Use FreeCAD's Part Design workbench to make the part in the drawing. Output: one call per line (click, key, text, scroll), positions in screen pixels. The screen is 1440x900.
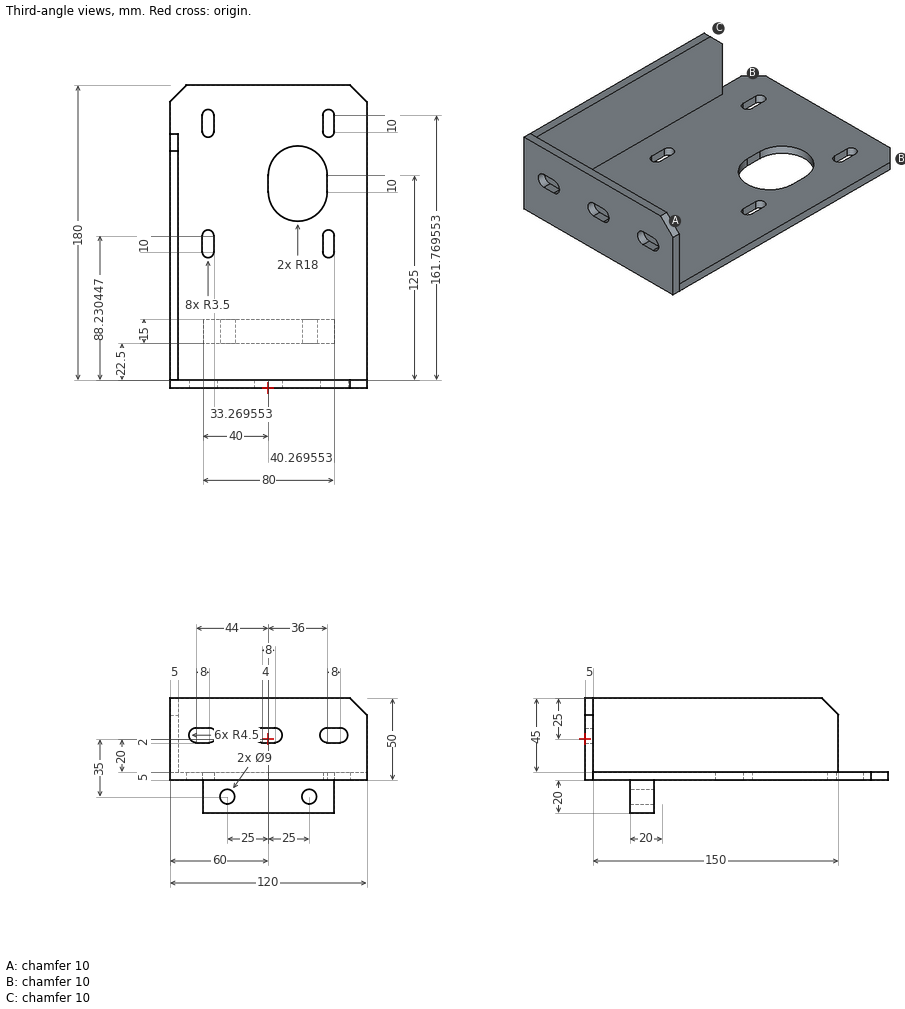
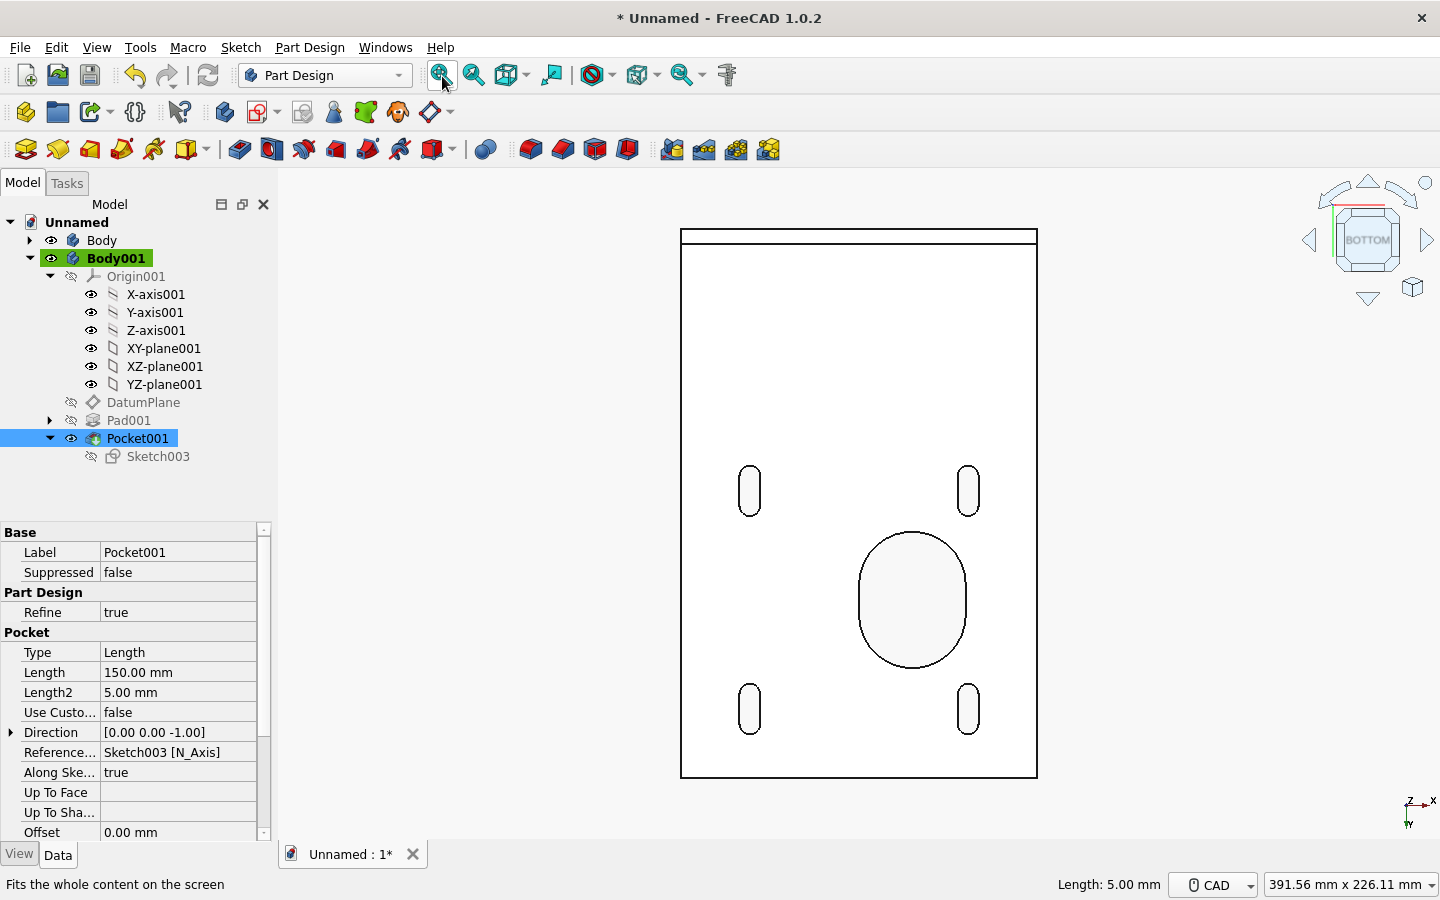
scroll(681, 777, up, 5)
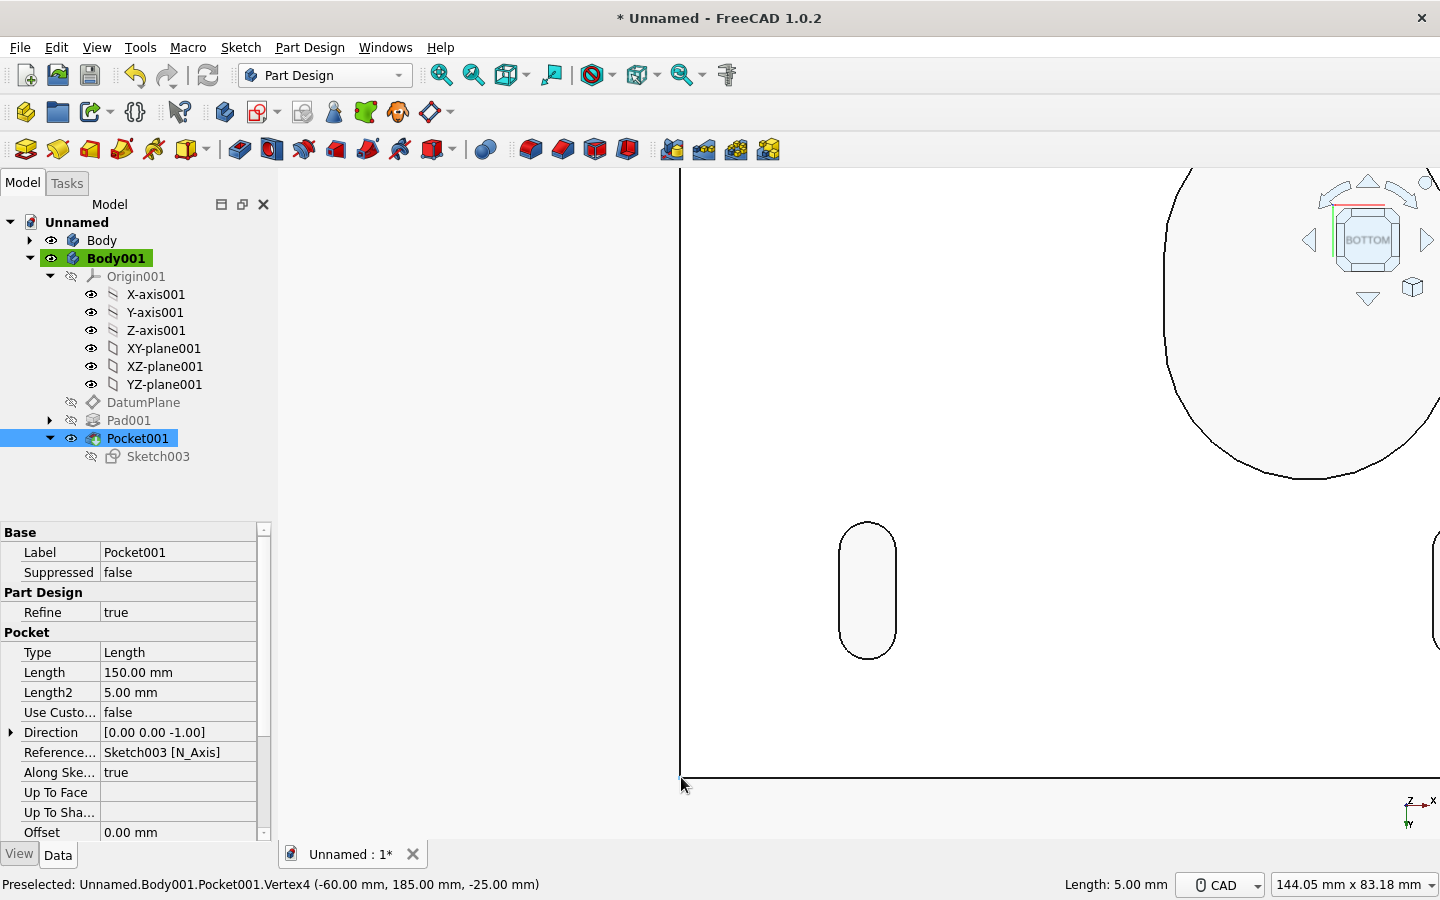
key(v)
key(f)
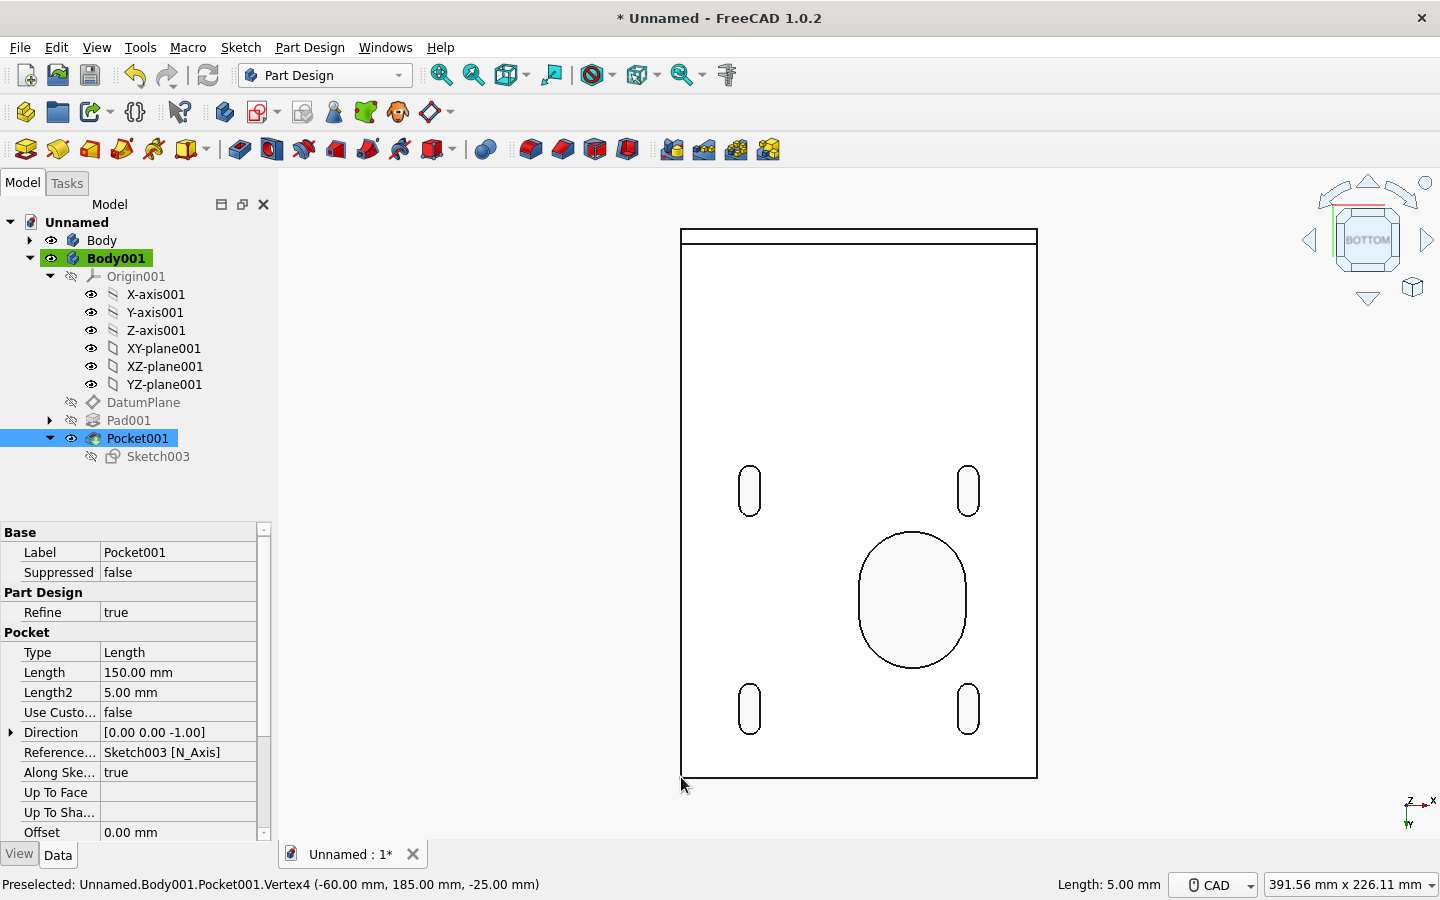
key(4)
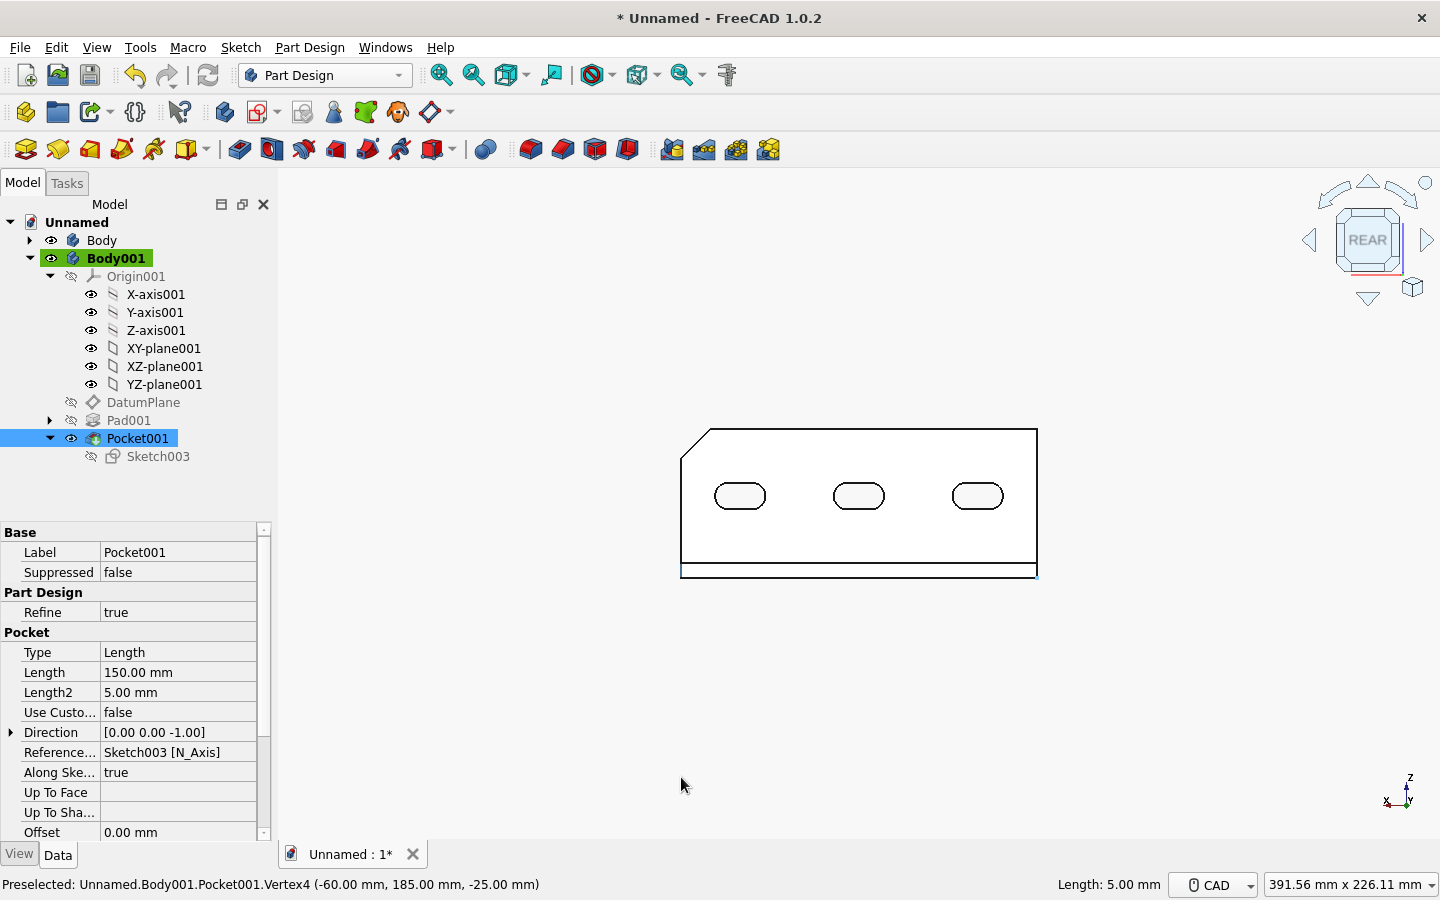
click(442, 76)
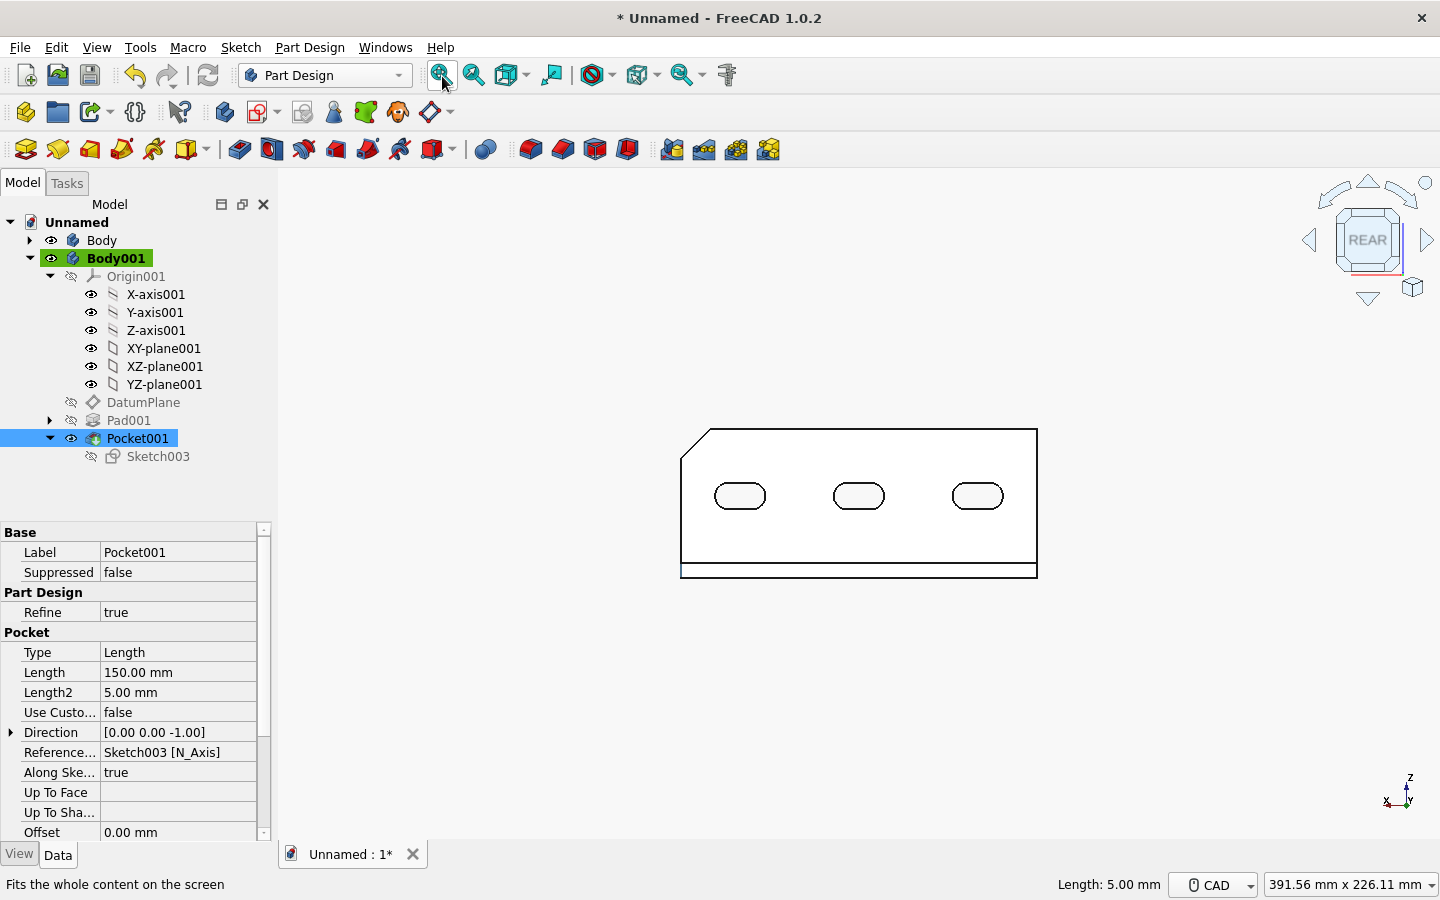
click(1037, 569, ctrl)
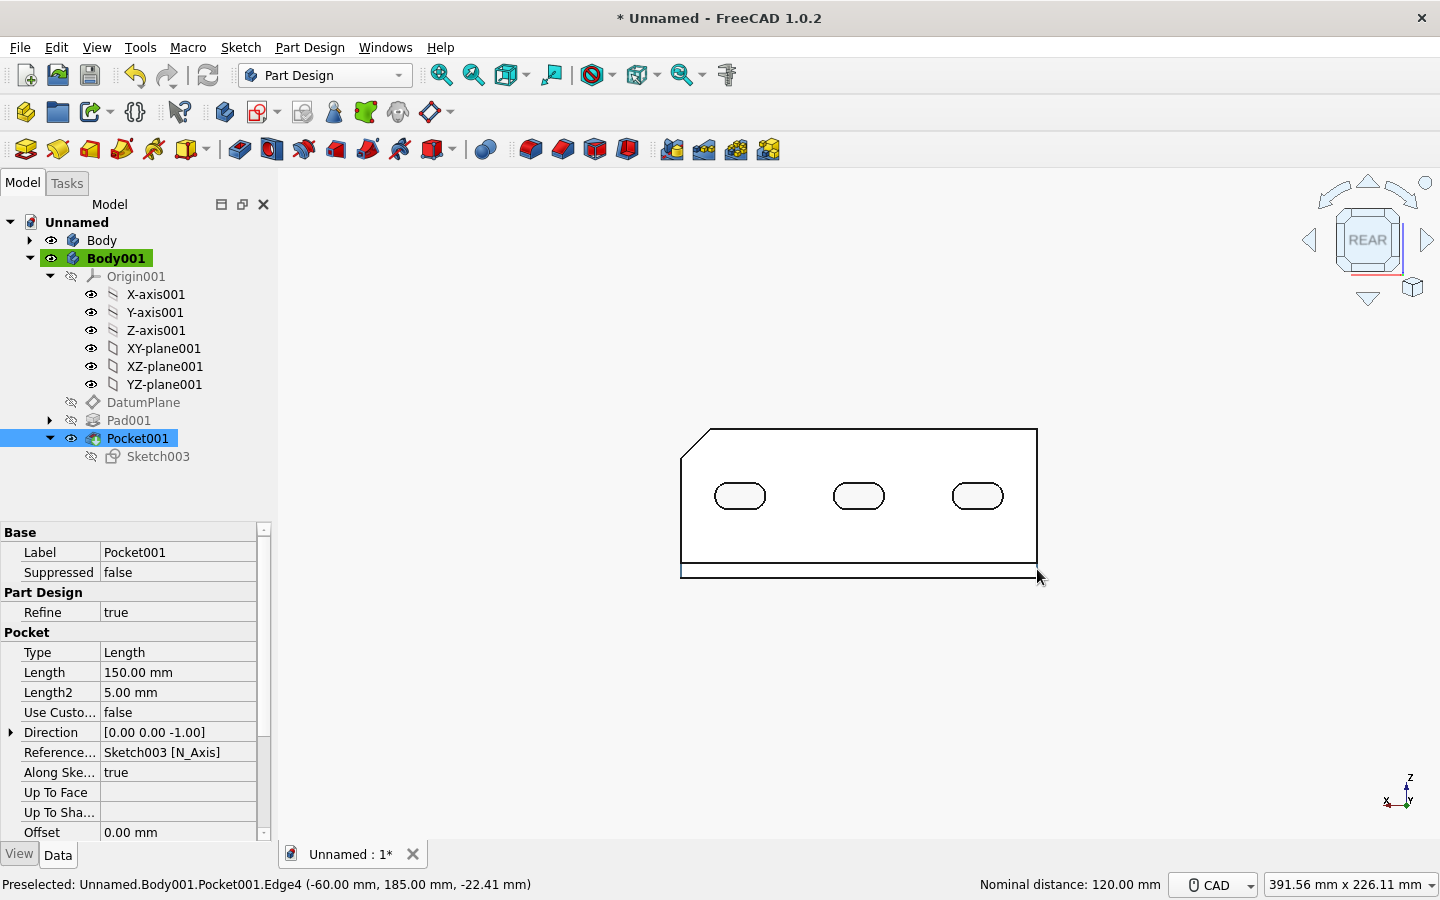
click(564, 150)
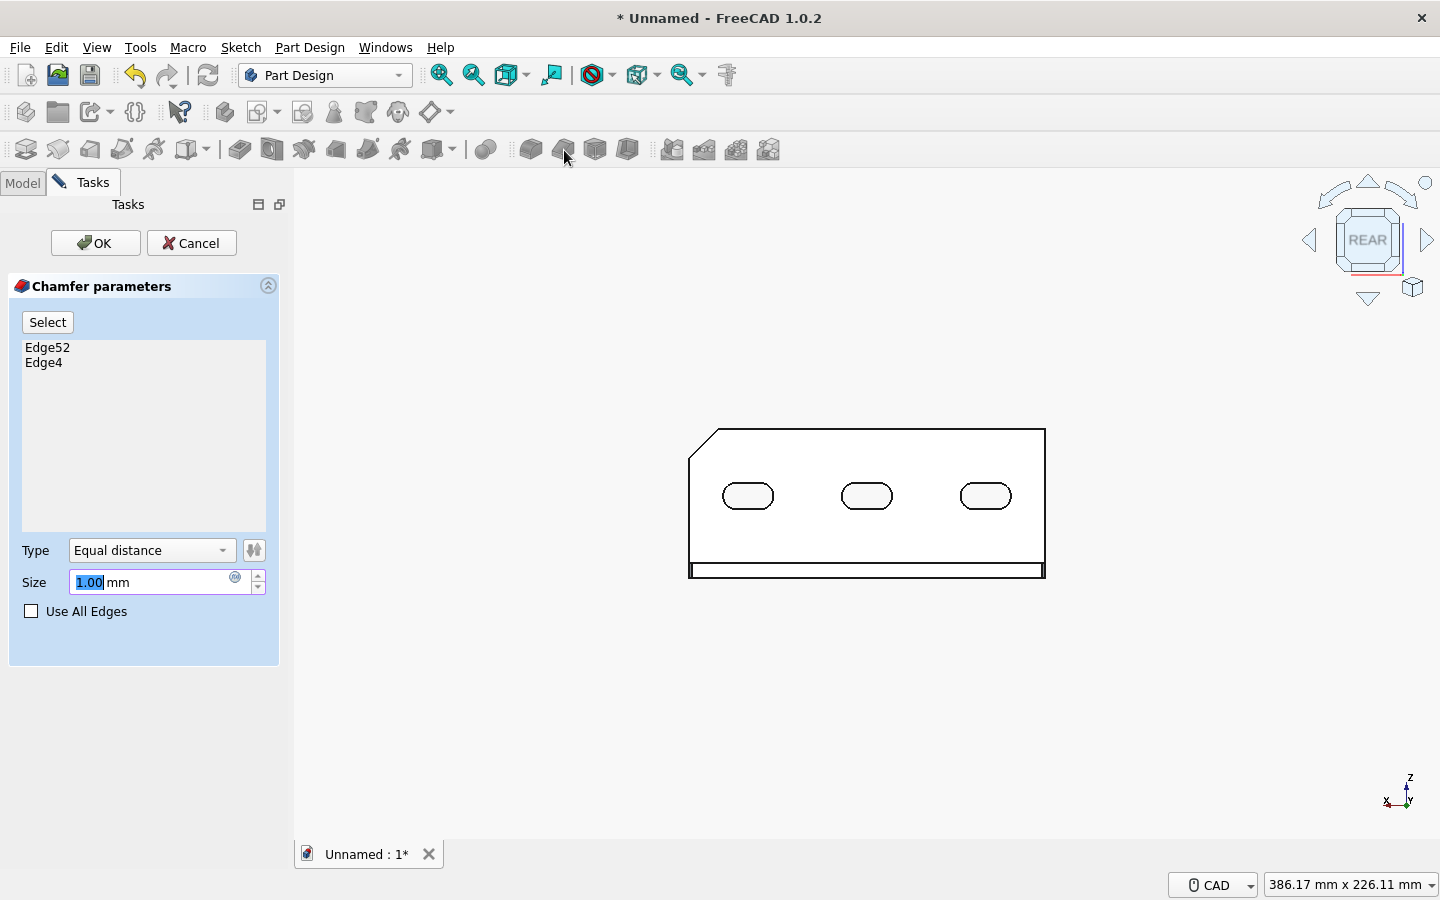
text(10)
key(Tab)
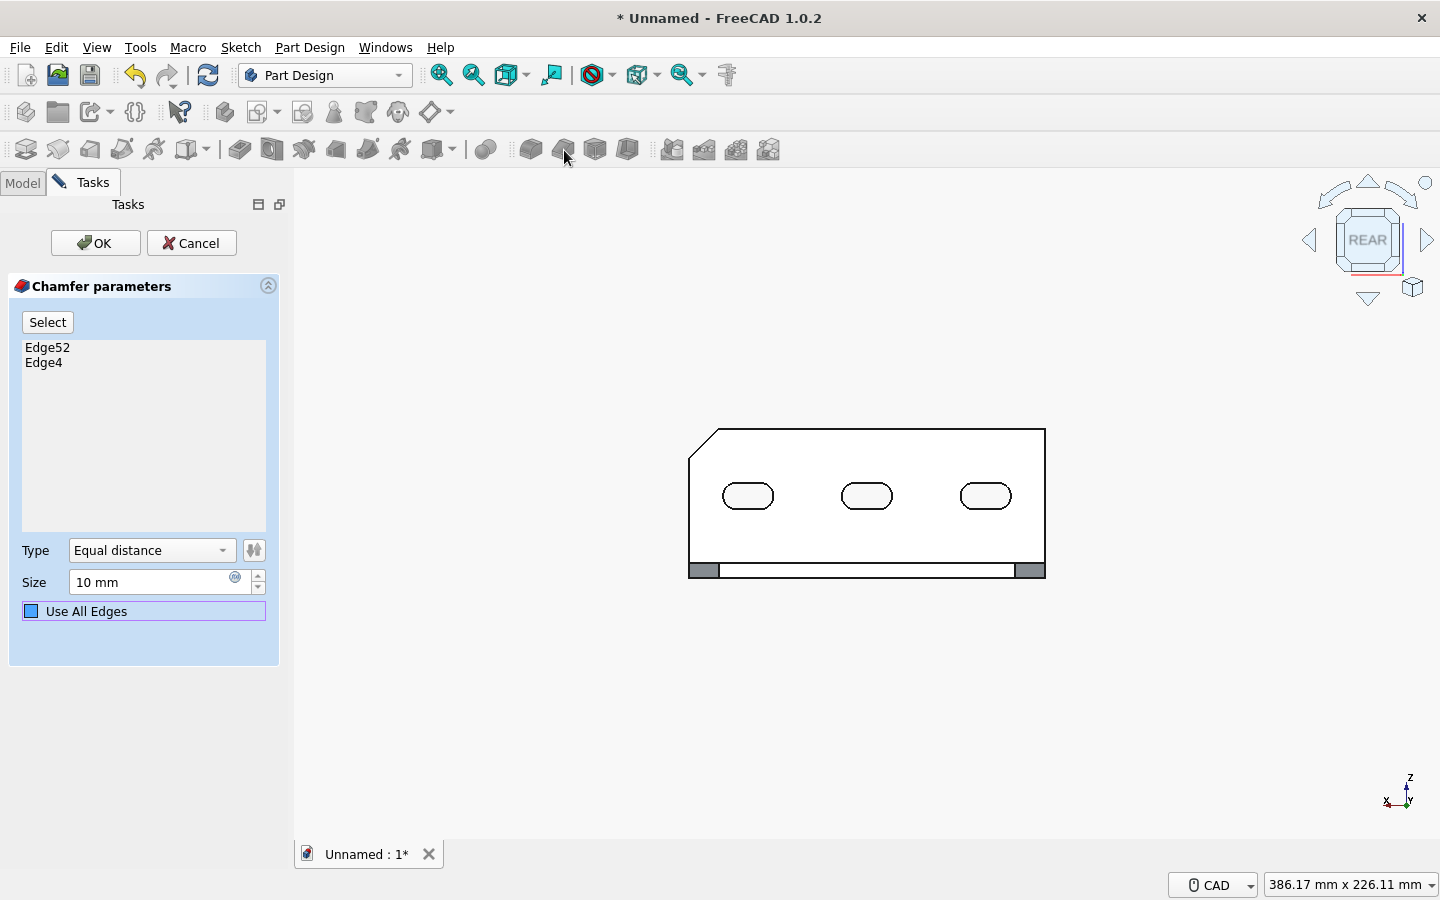
click(96, 243)